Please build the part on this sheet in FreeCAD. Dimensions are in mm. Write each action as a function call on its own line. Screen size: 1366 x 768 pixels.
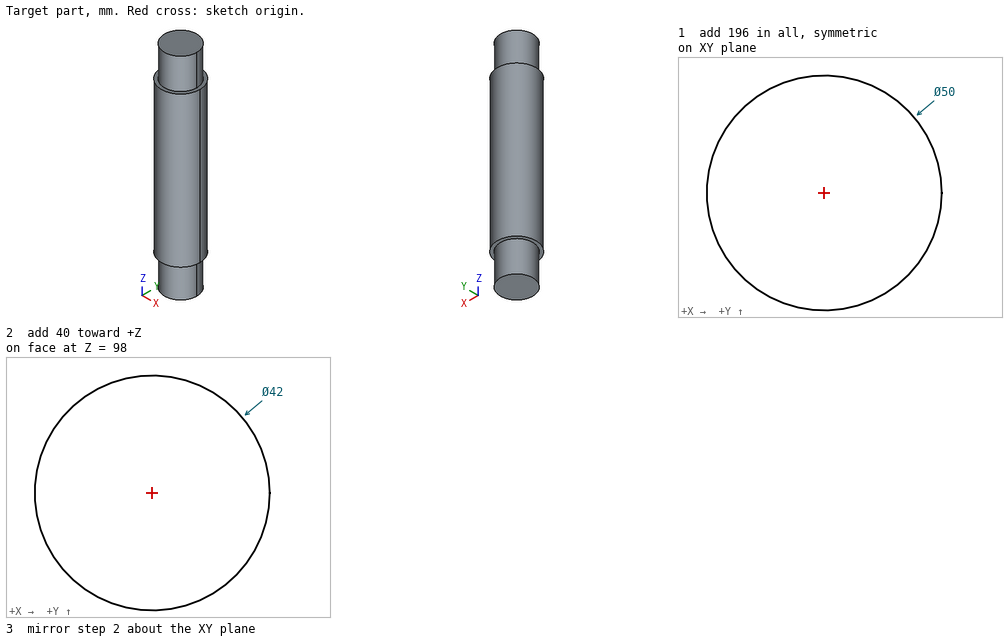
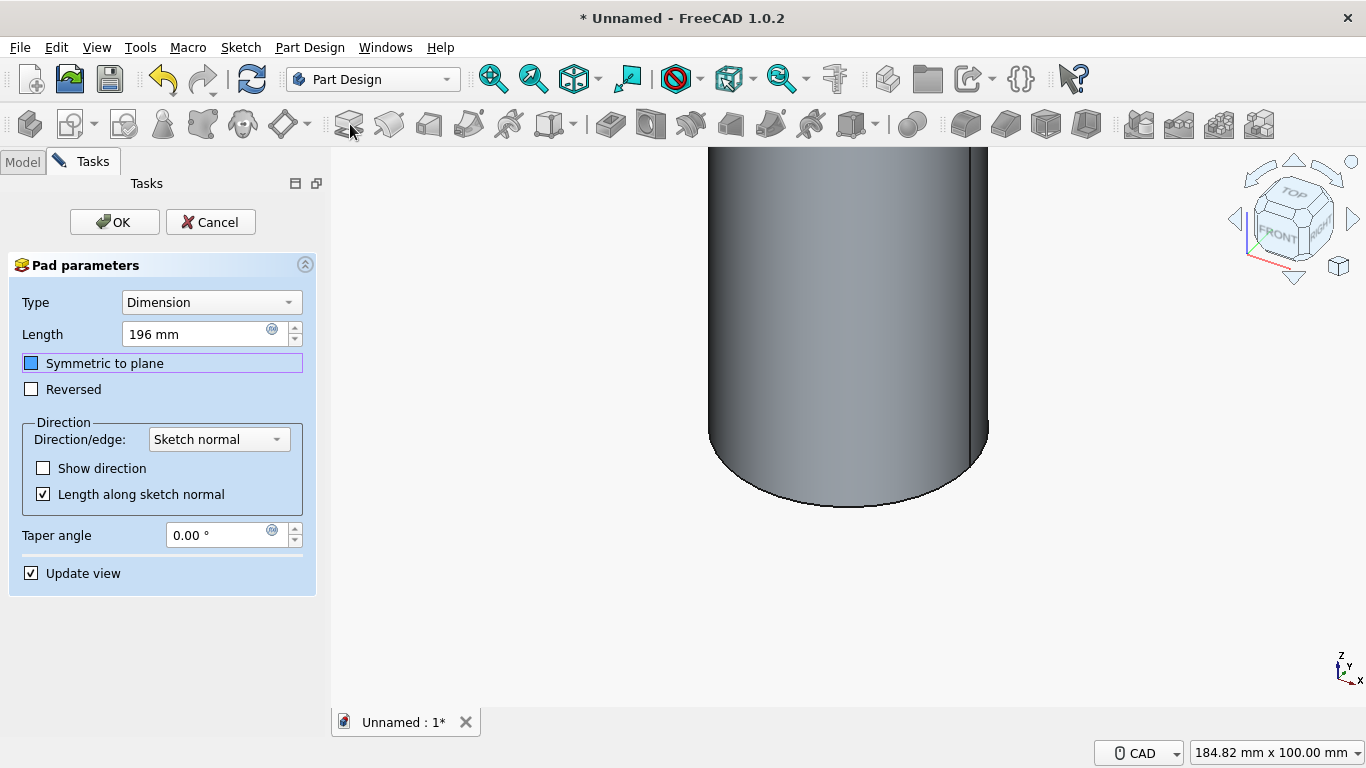
click(30, 363)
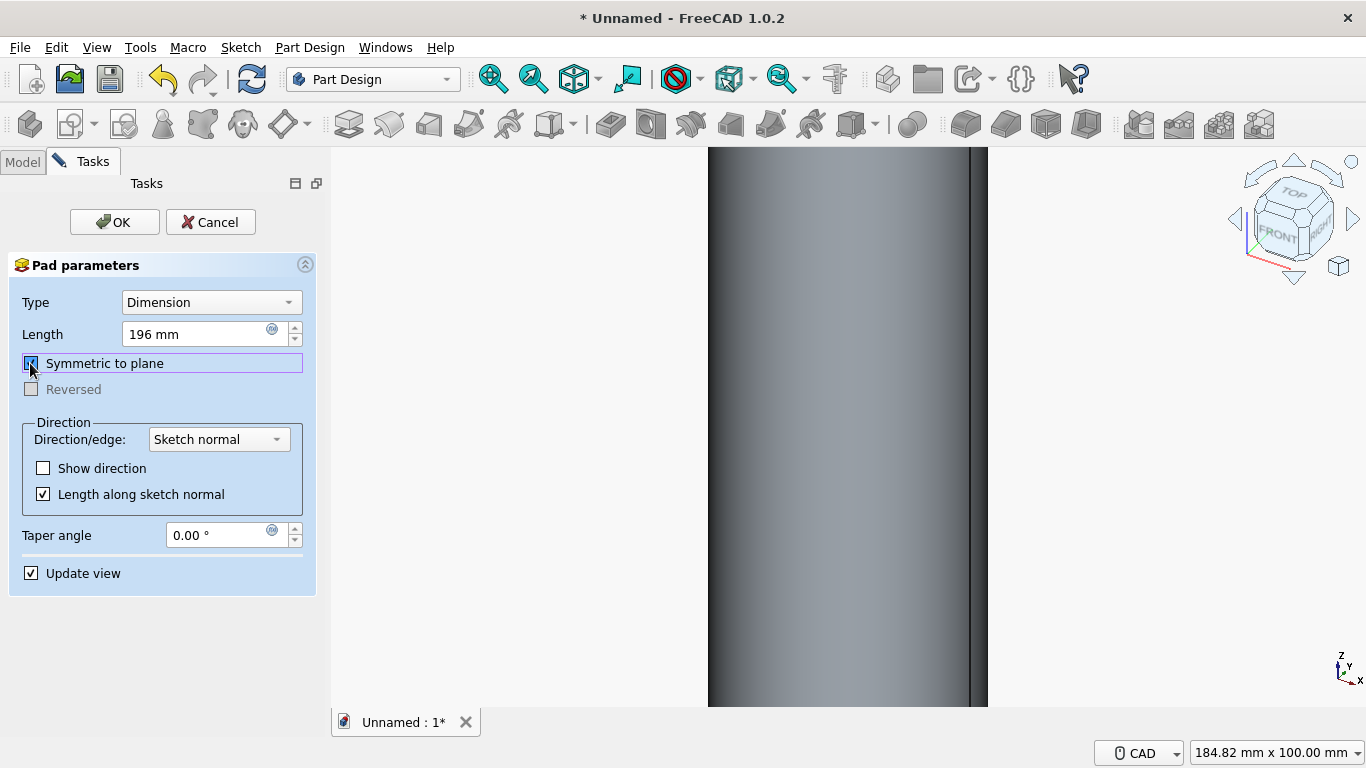
click(115, 222)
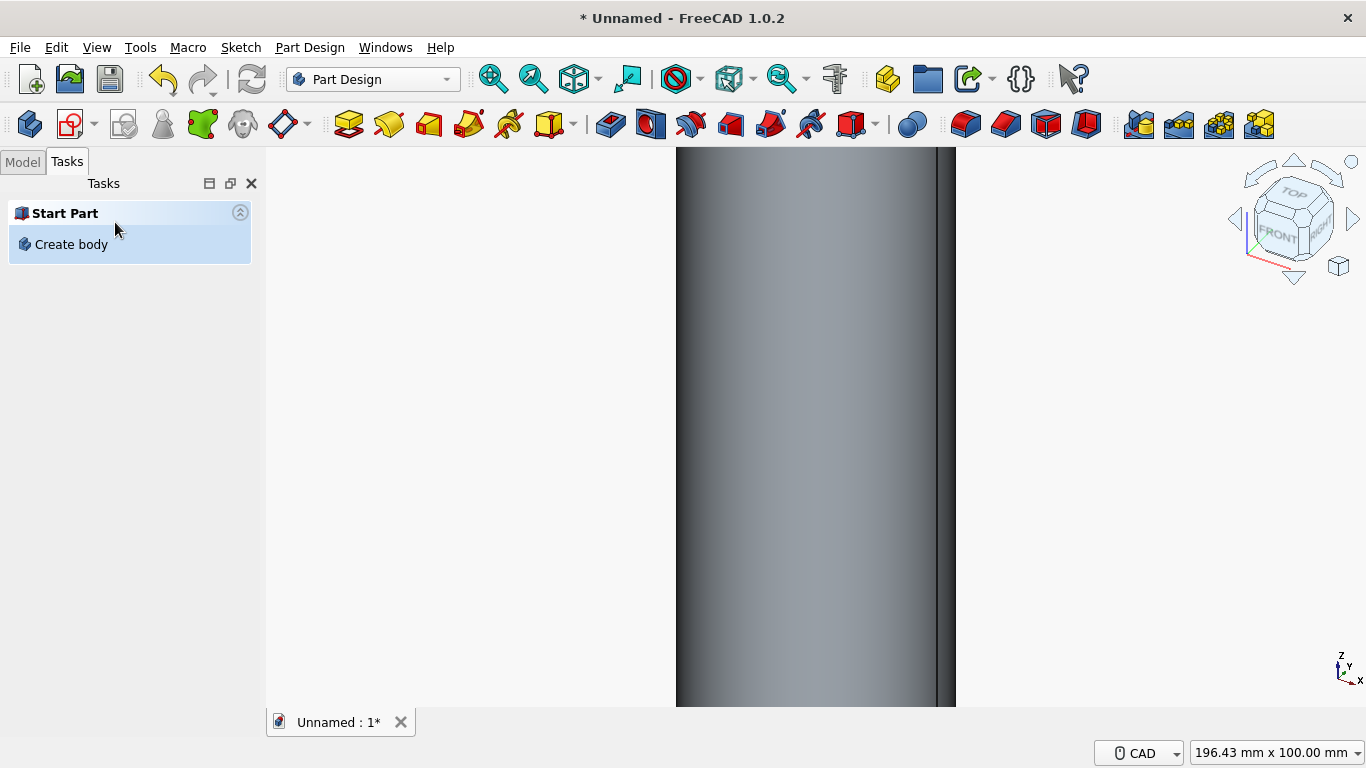
key(v)
key(f)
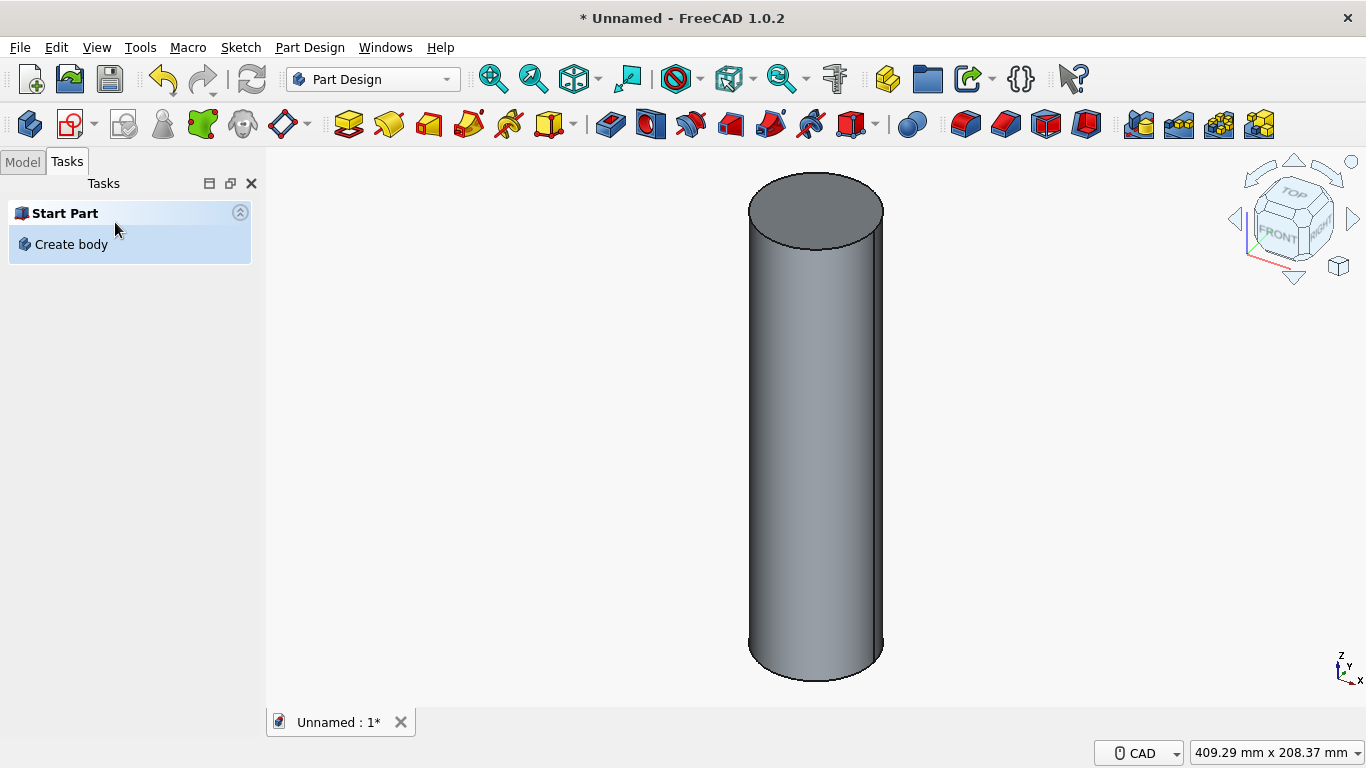
click(816, 210)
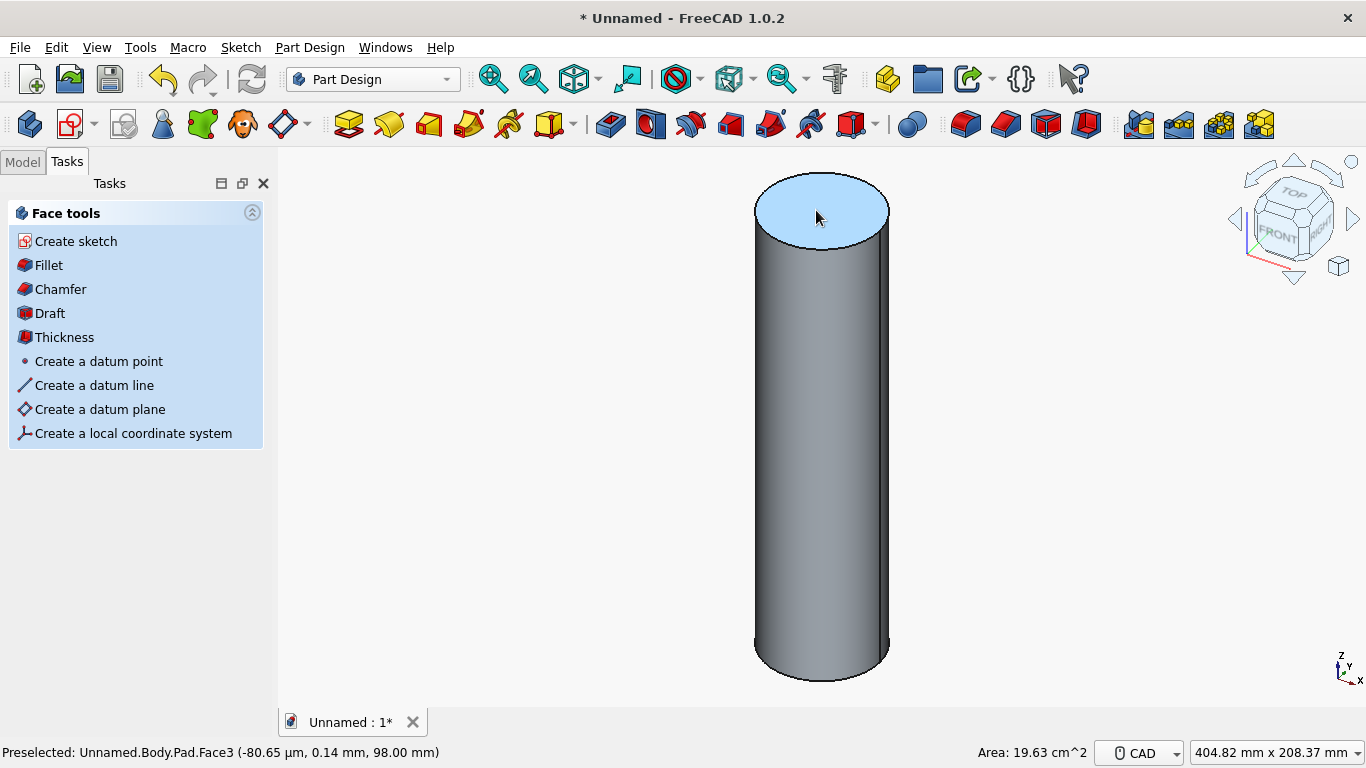
click(70, 124)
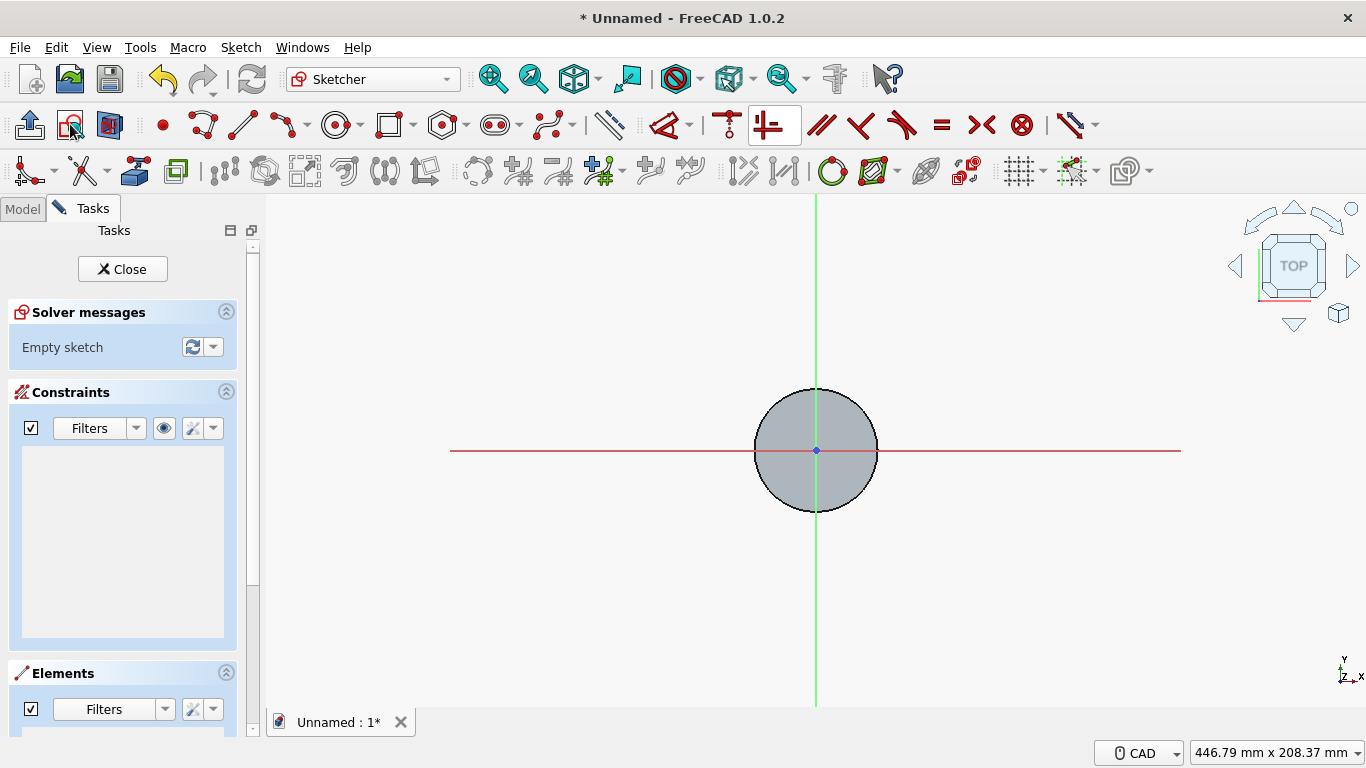
scroll(846, 450, up, 6)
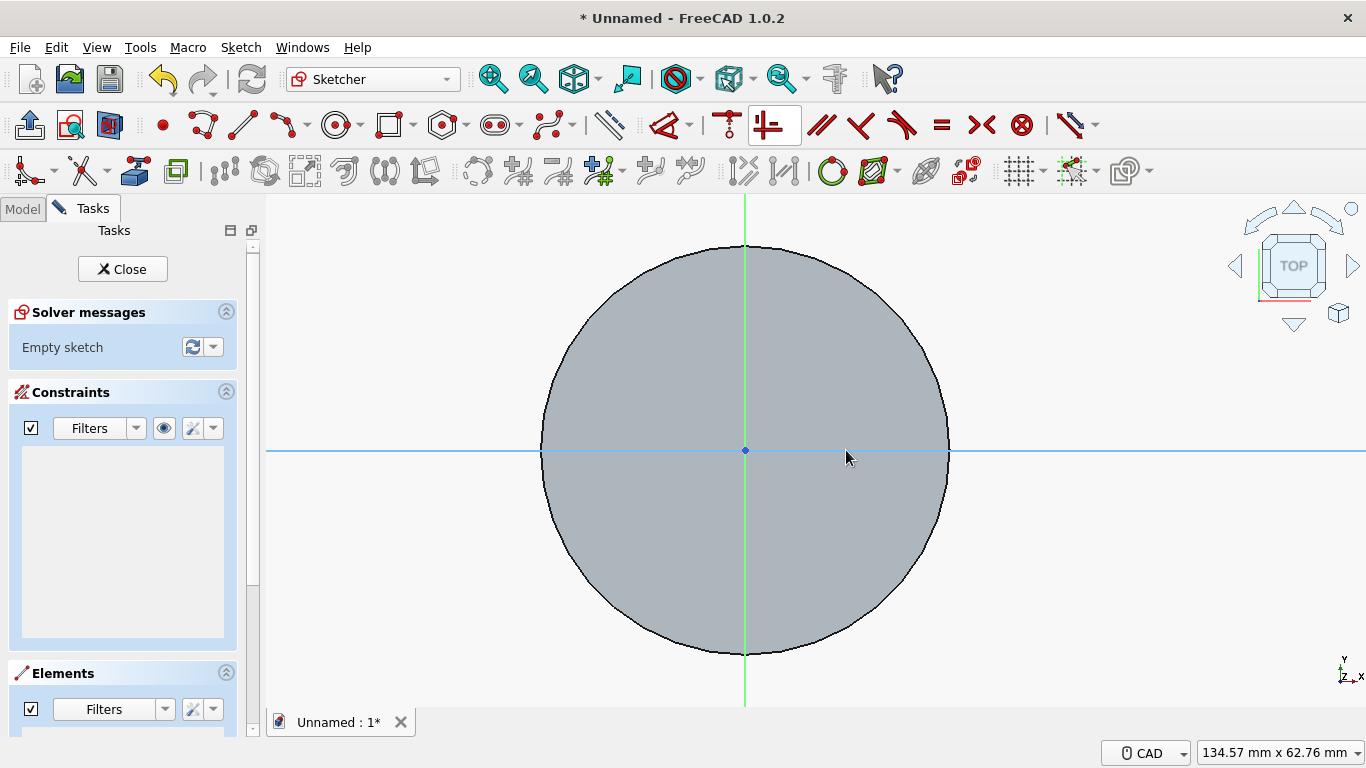
key(g)
key(c)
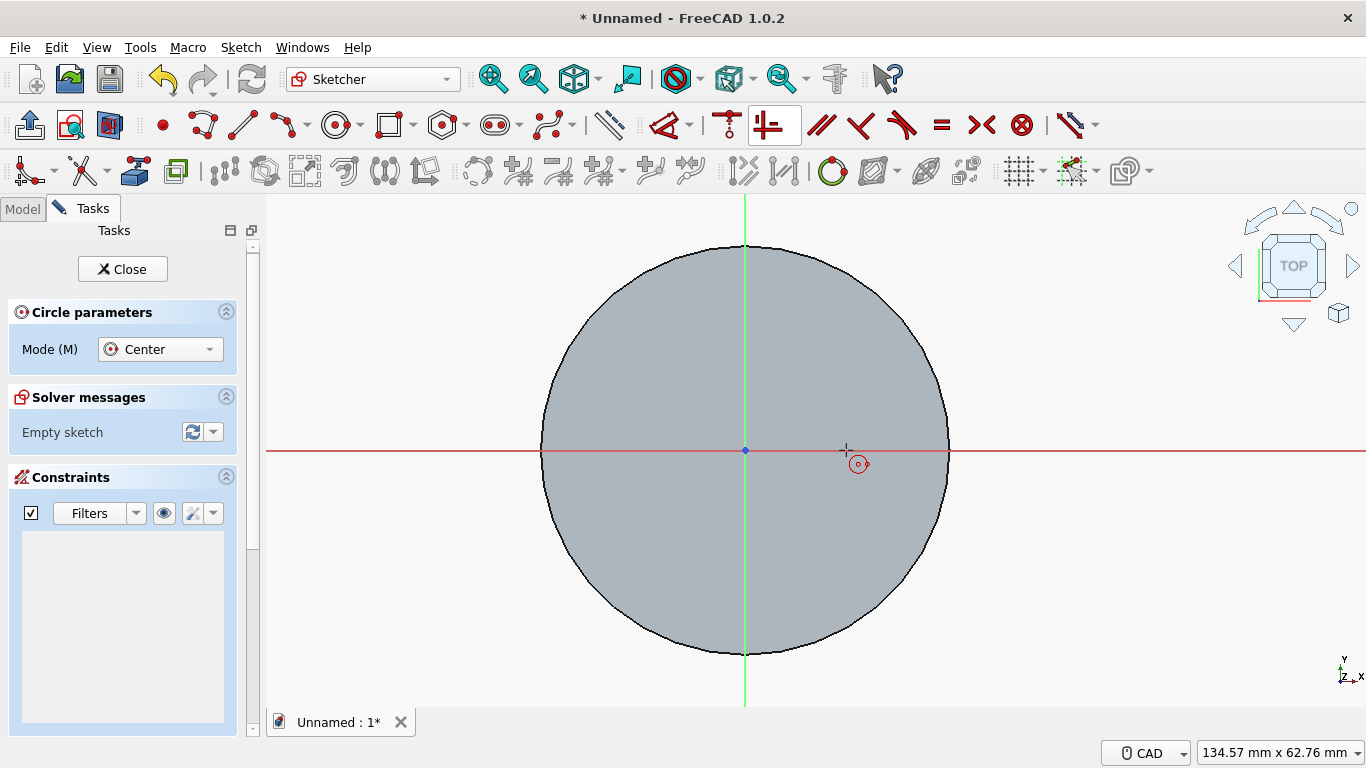
click(745, 450)
move(867, 329)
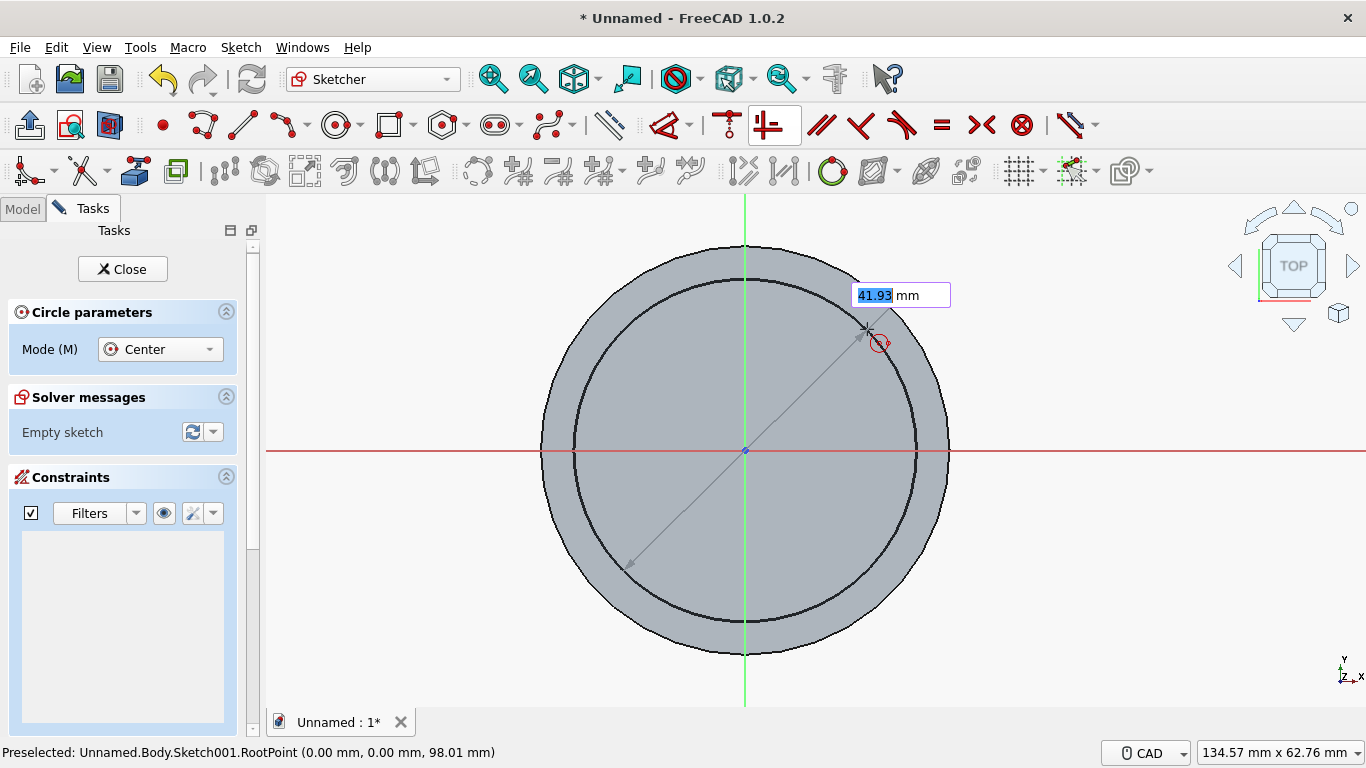
text(42)
key(Return)
key(Escape)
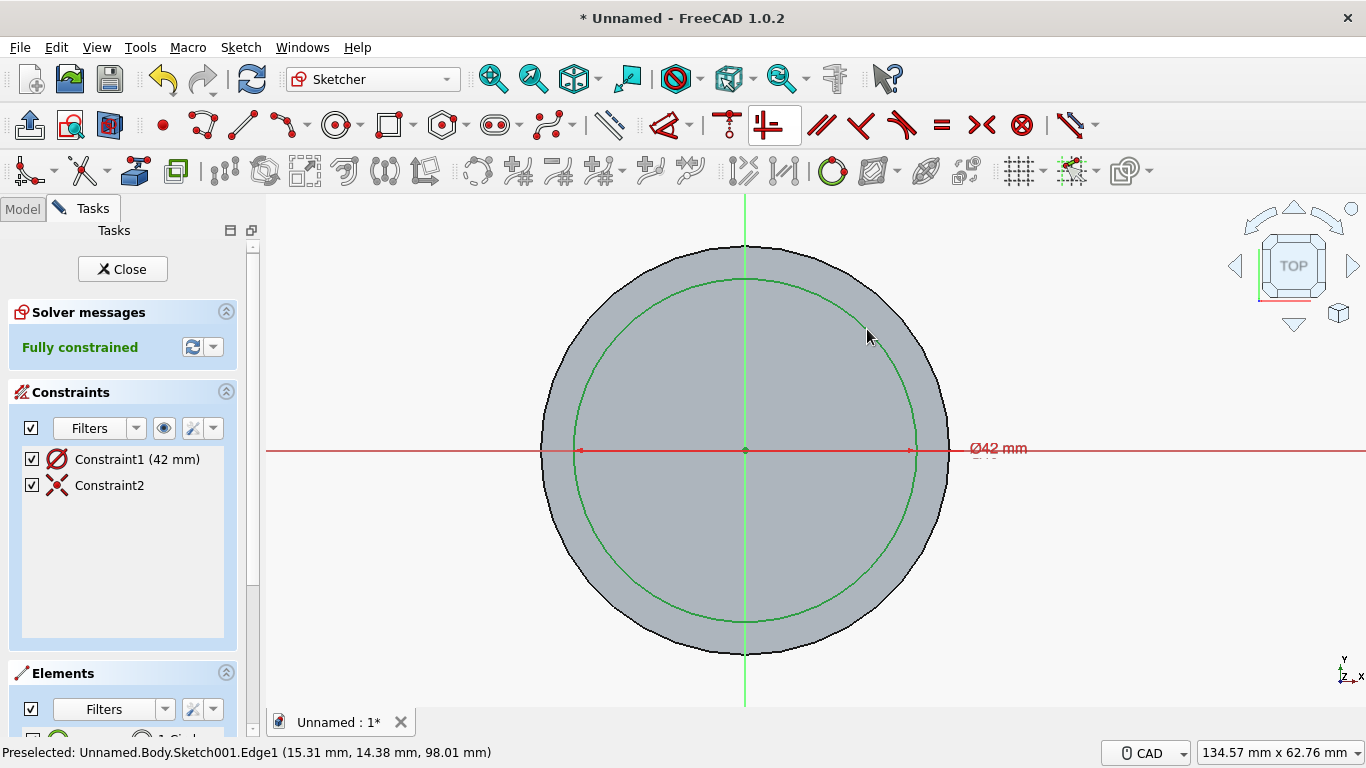
click(123, 269)